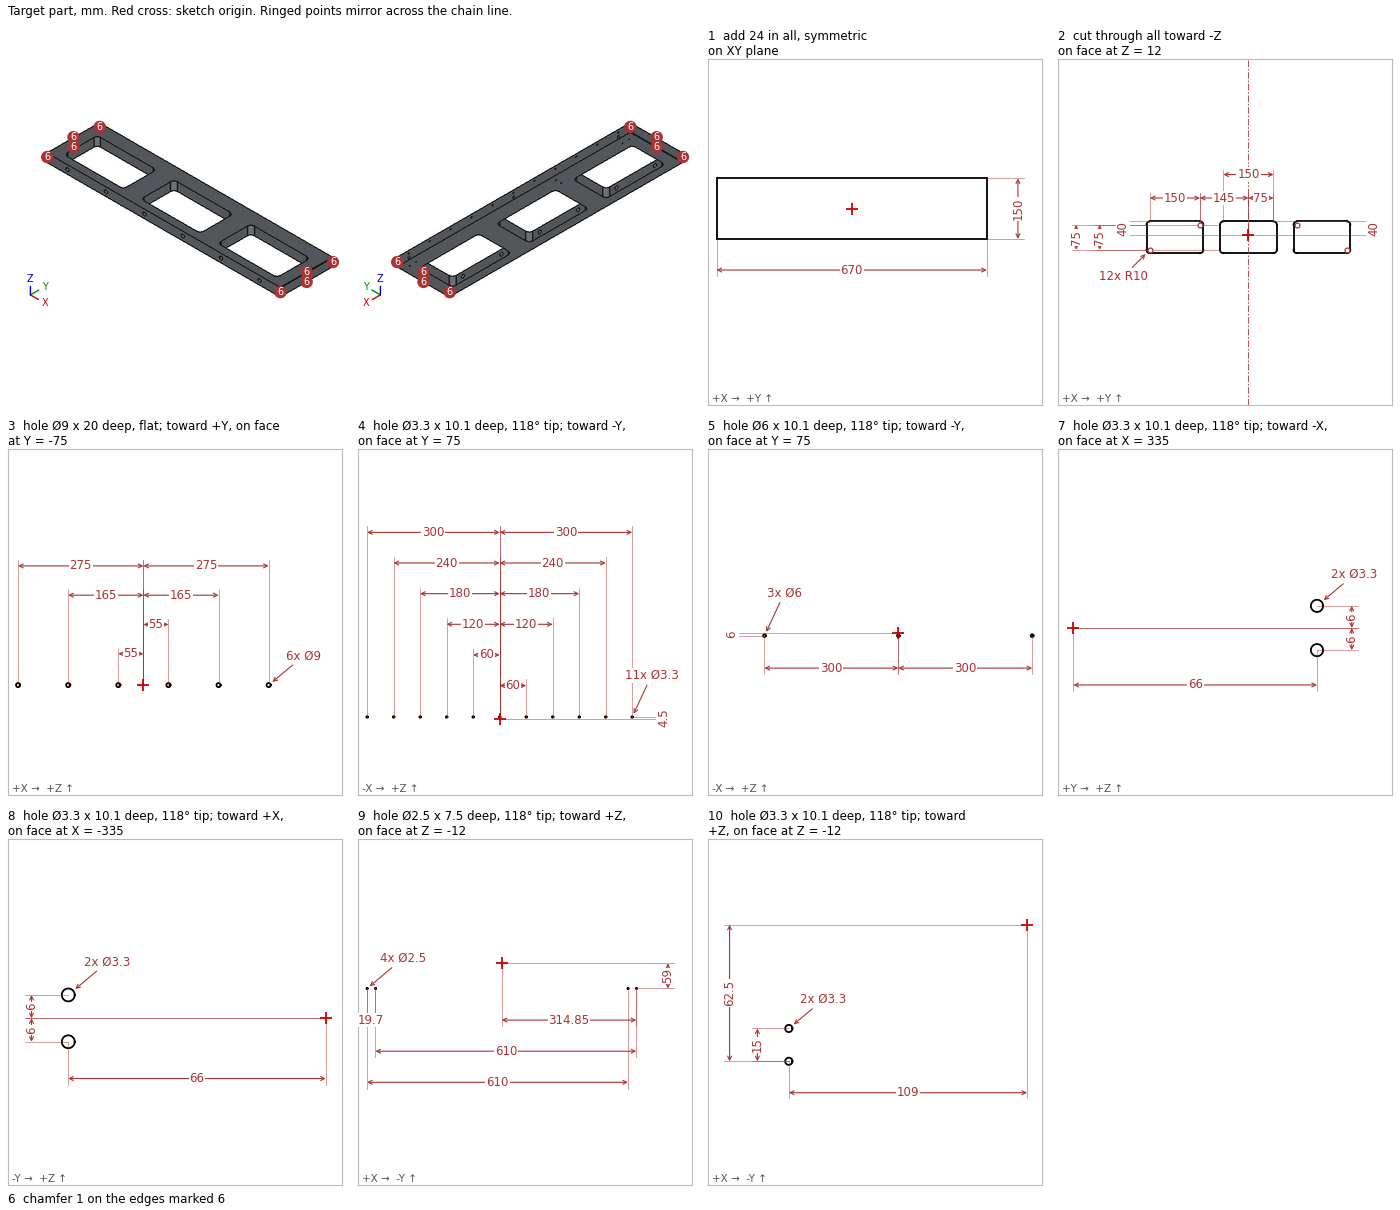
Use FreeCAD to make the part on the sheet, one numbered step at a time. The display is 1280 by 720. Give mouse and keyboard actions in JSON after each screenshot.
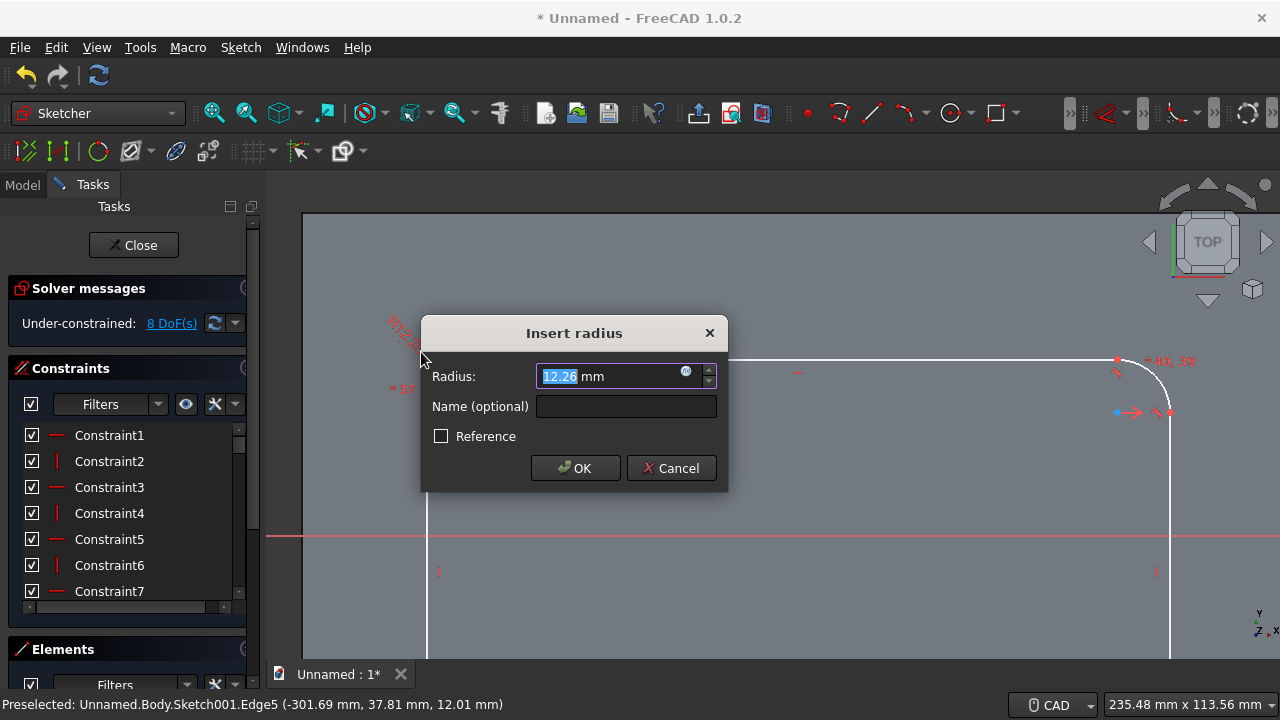
{"action": "type", "text": "10"}
{"action": "key", "text": "Return"}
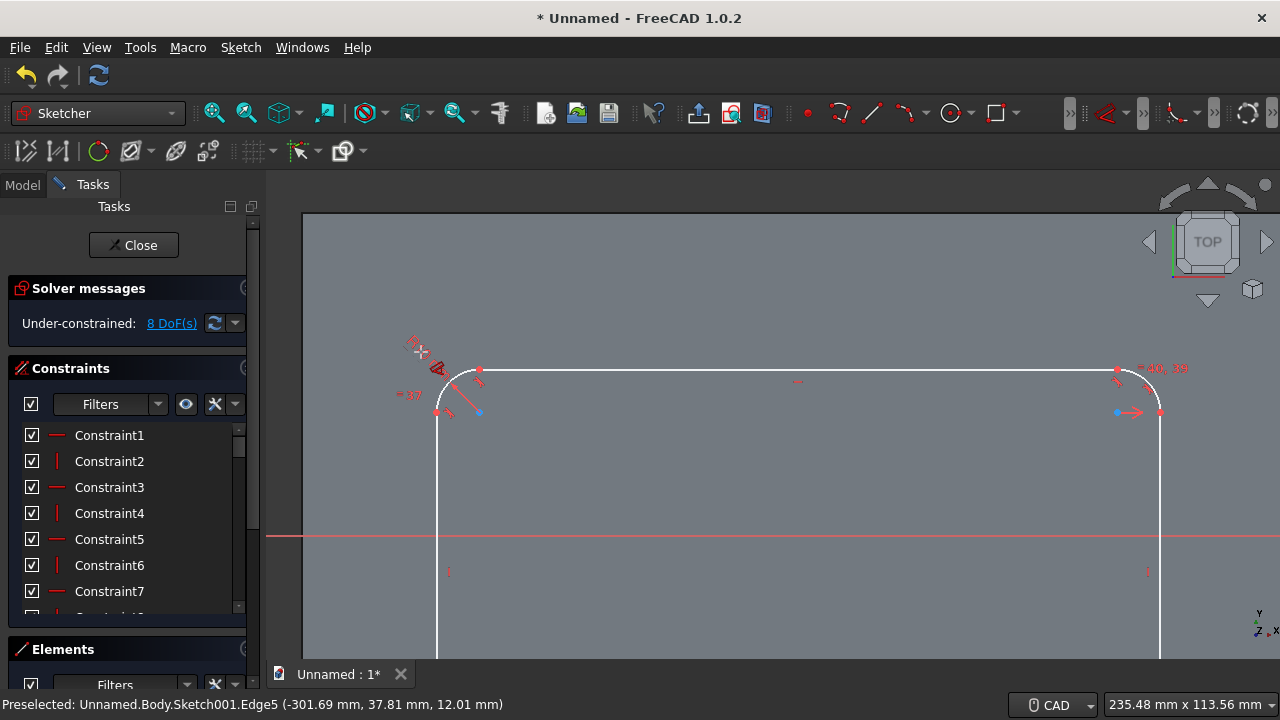
{"action": "left_click", "coordinate": [437, 508]}
{"action": "left_click", "coordinate": [403, 522]}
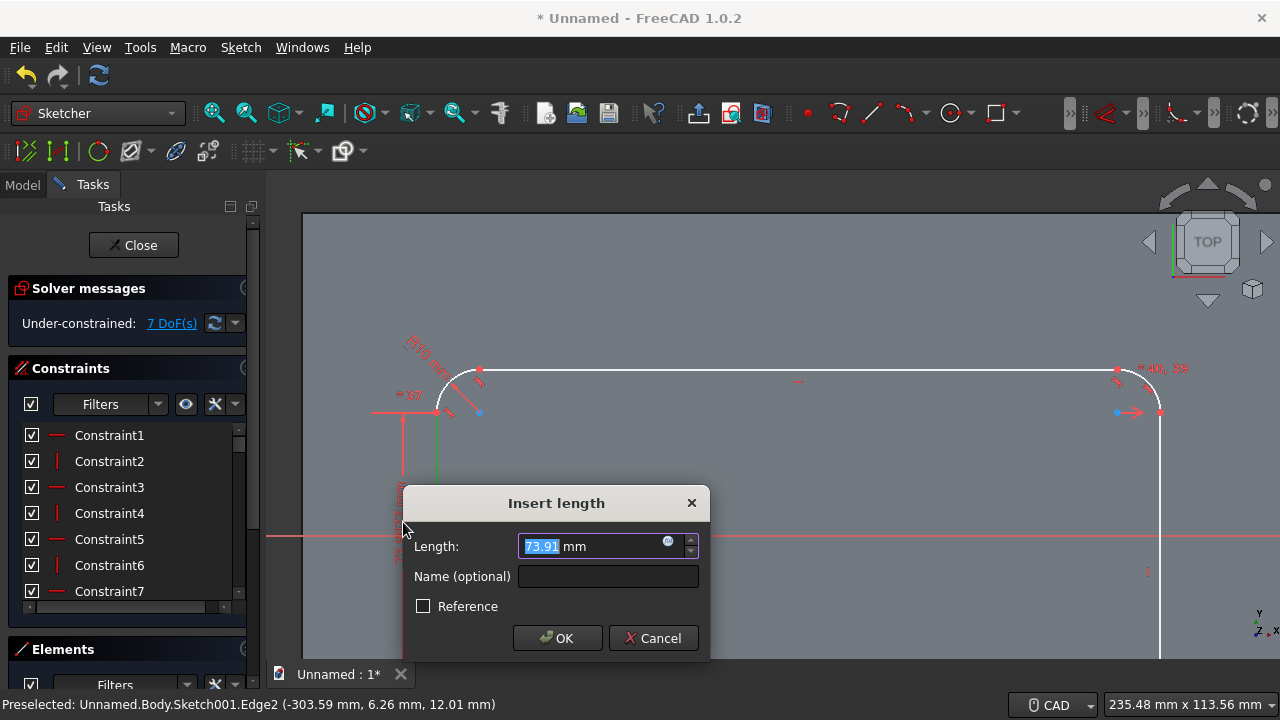
{"action": "type", "text": "75"}
{"action": "key", "text": "Return"}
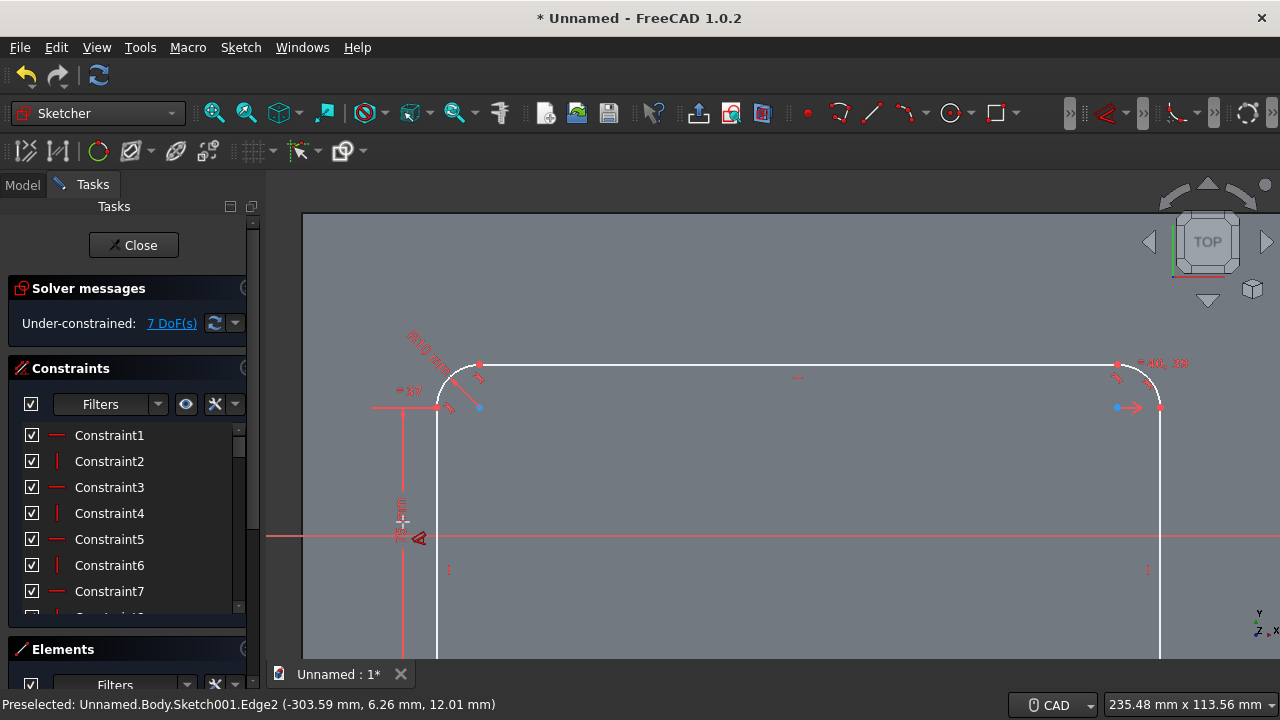
{"action": "scroll", "coordinate": [442, 376], "scroll_direction": "down", "scroll_amount": 8}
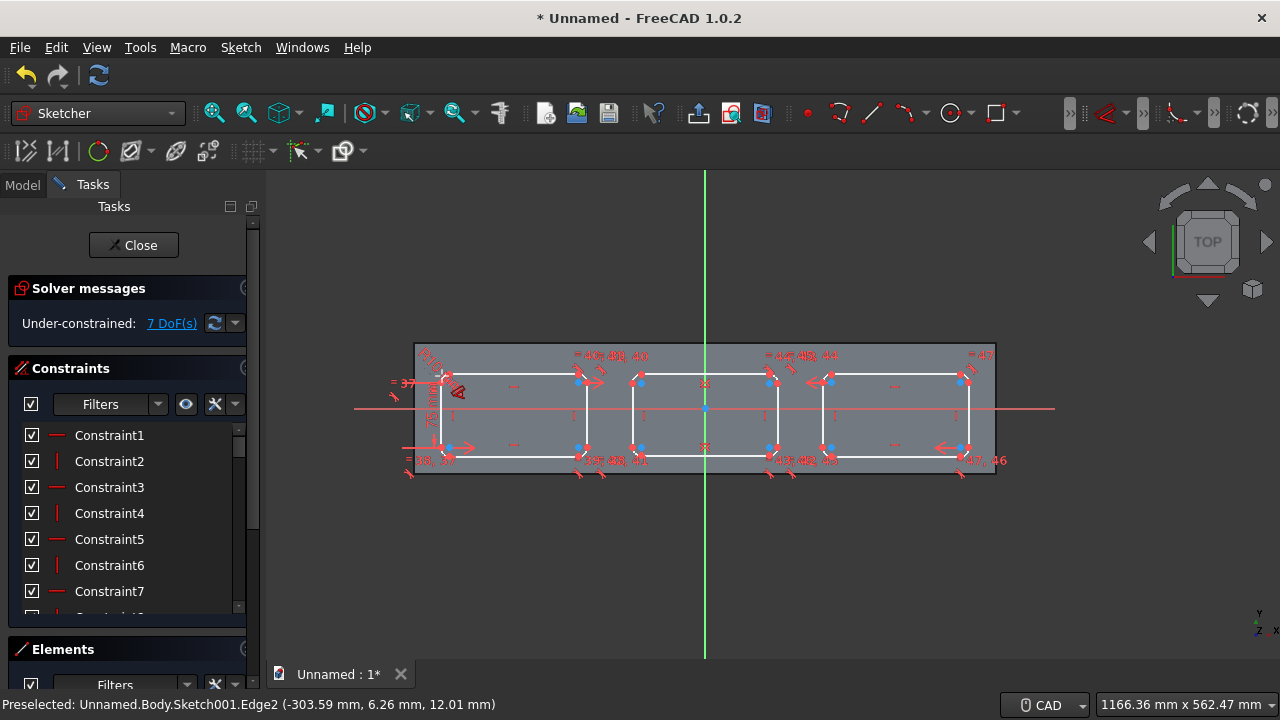
{"action": "scroll", "coordinate": [633, 402], "scroll_direction": "up", "scroll_amount": 4}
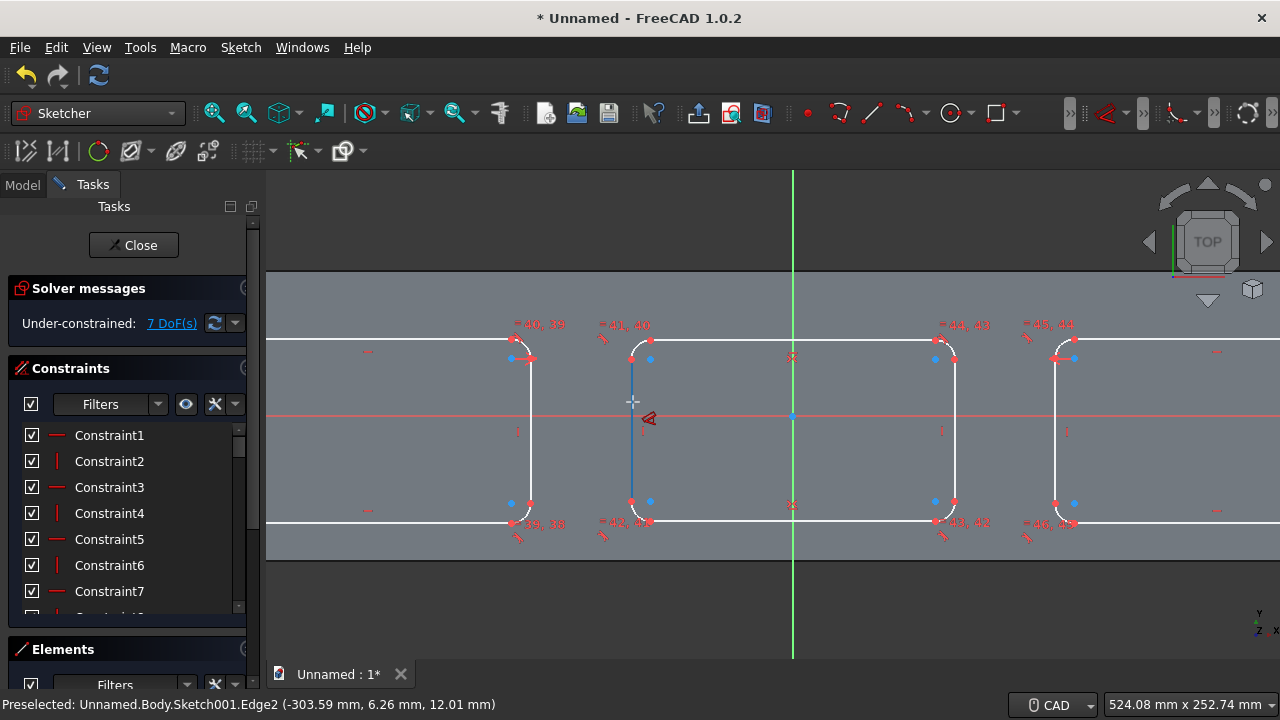
{"action": "left_click", "coordinate": [632, 402]}
{"action": "left_click", "coordinate": [598, 431]}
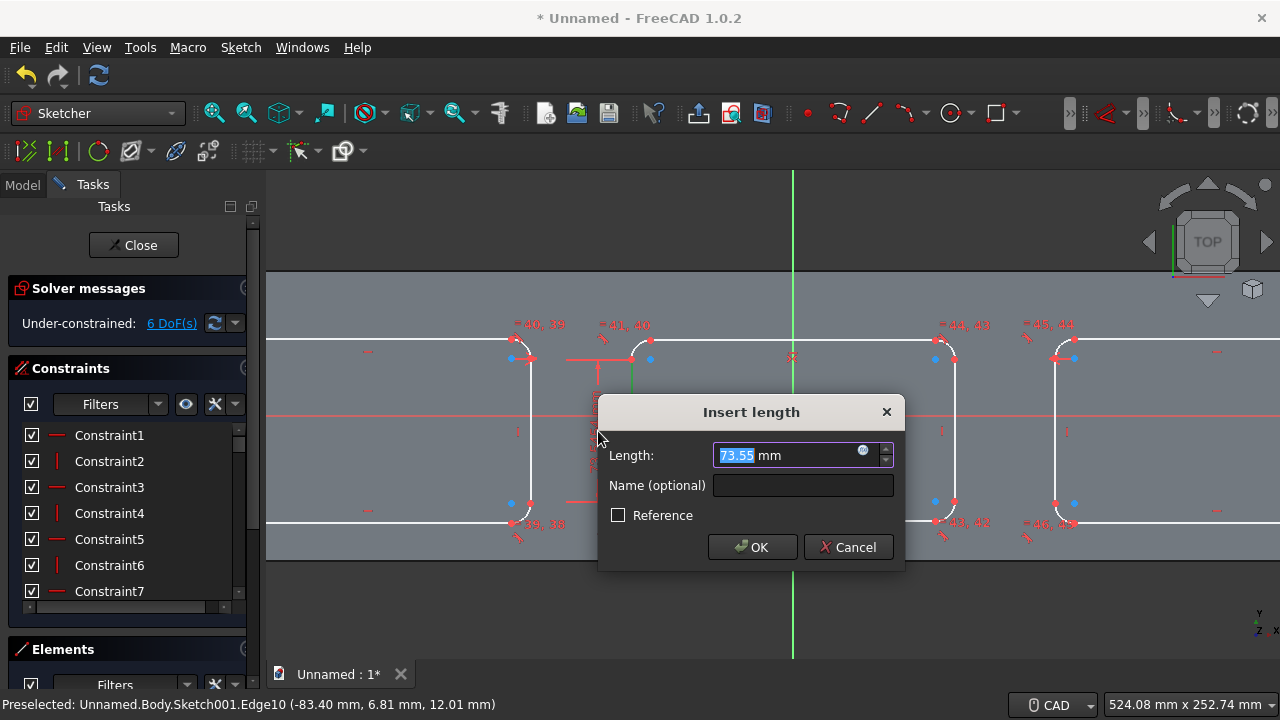
{"action": "type", "text": "75"}
{"action": "key", "text": "Return"}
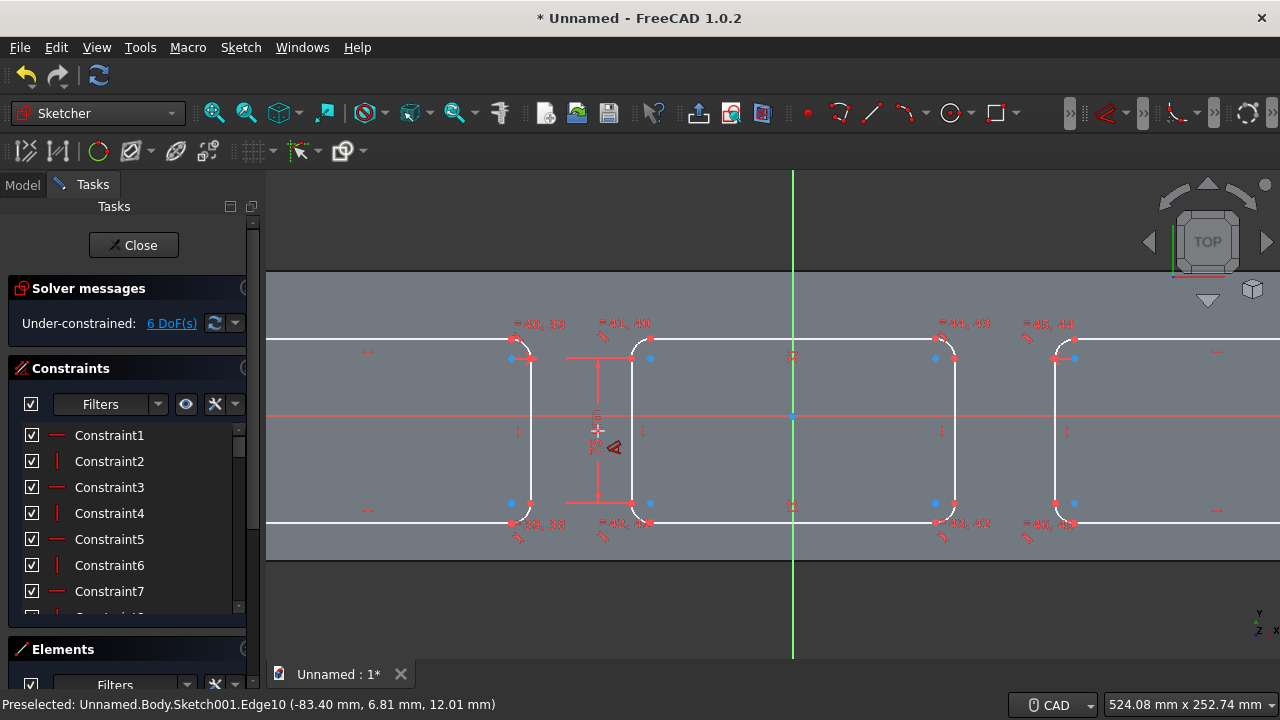
{"action": "left_click", "coordinate": [425, 339]}
{"action": "left_click", "coordinate": [403, 305]}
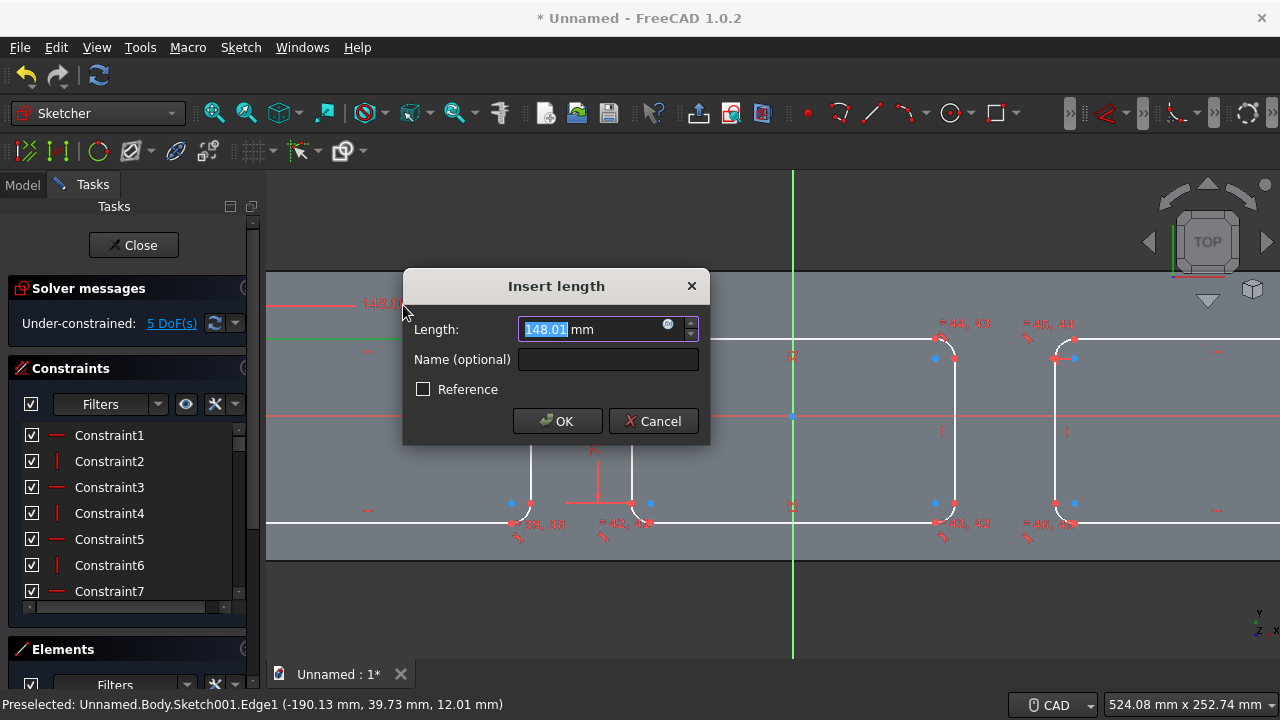
{"action": "type", "text": "150"}
{"action": "key", "text": "Return"}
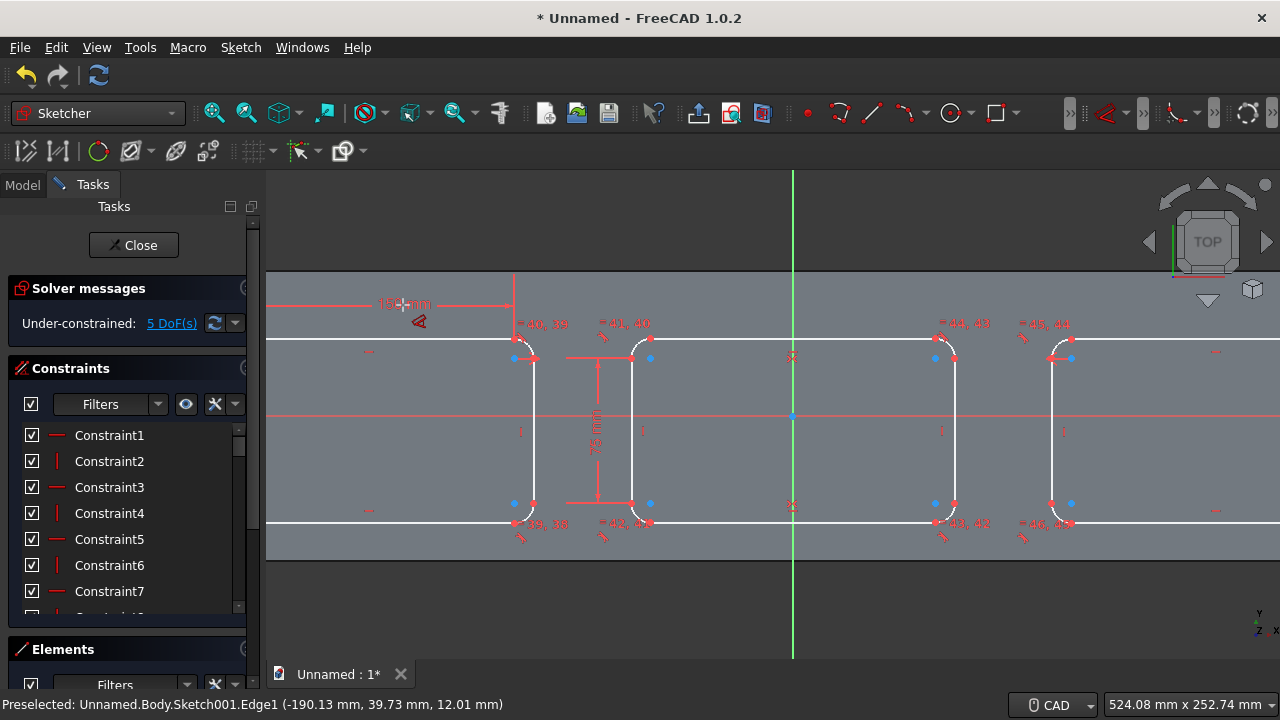
{"action": "left_click", "coordinate": [850, 339]}
{"action": "left_click", "coordinate": [728, 305]}